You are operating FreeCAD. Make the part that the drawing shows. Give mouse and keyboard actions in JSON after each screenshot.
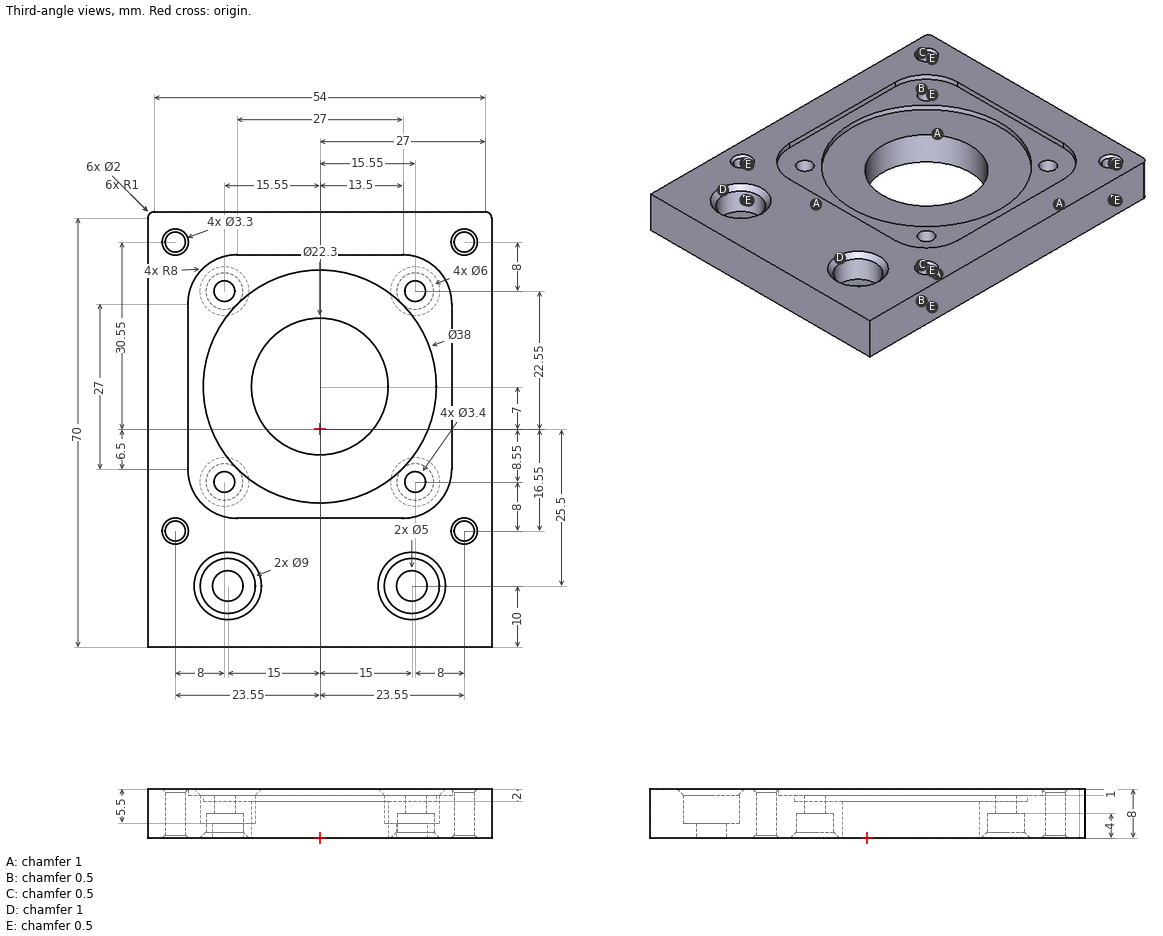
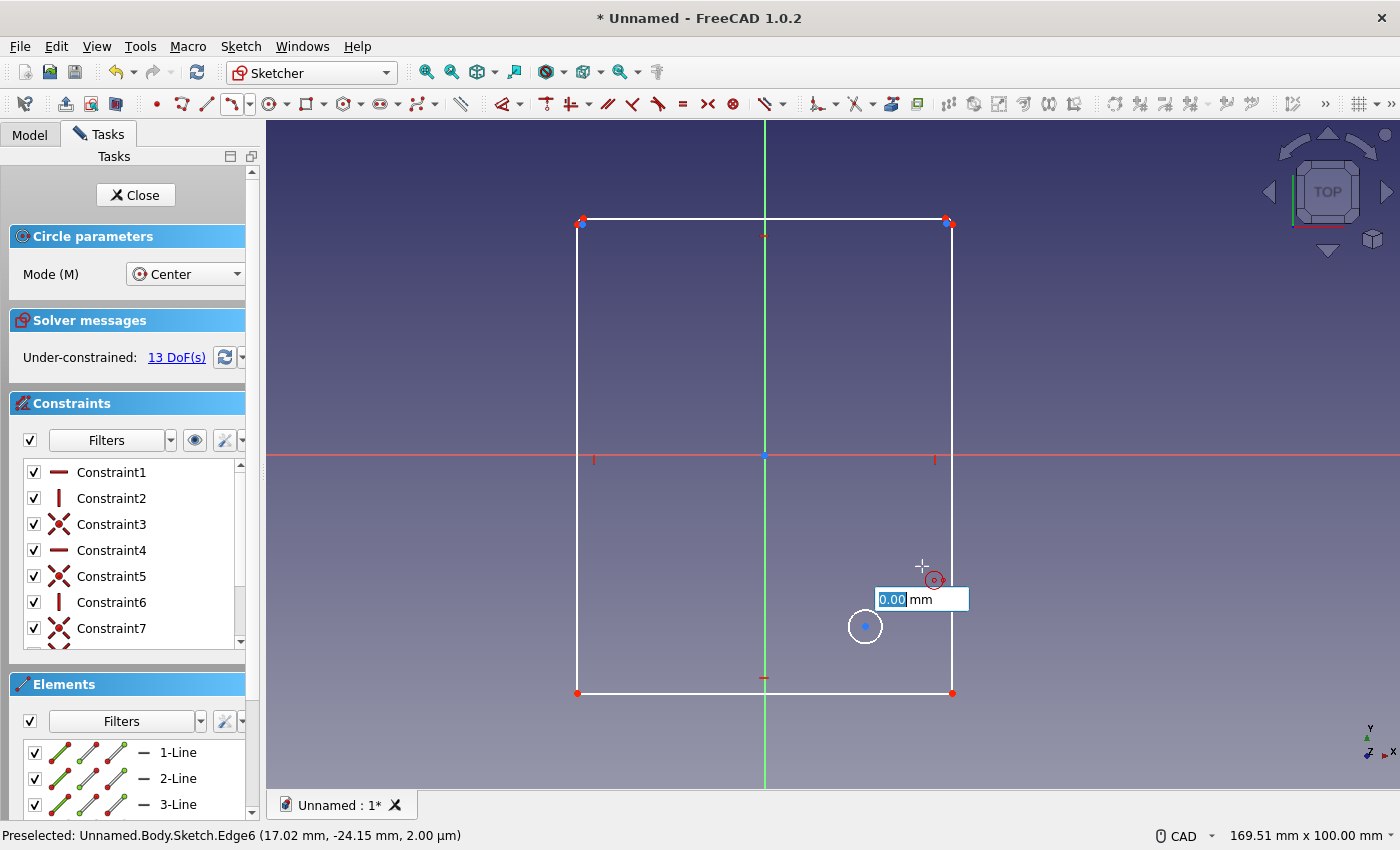
{"action": "scroll", "coordinate": [927, 561], "scroll_direction": "up", "scroll_amount": 5}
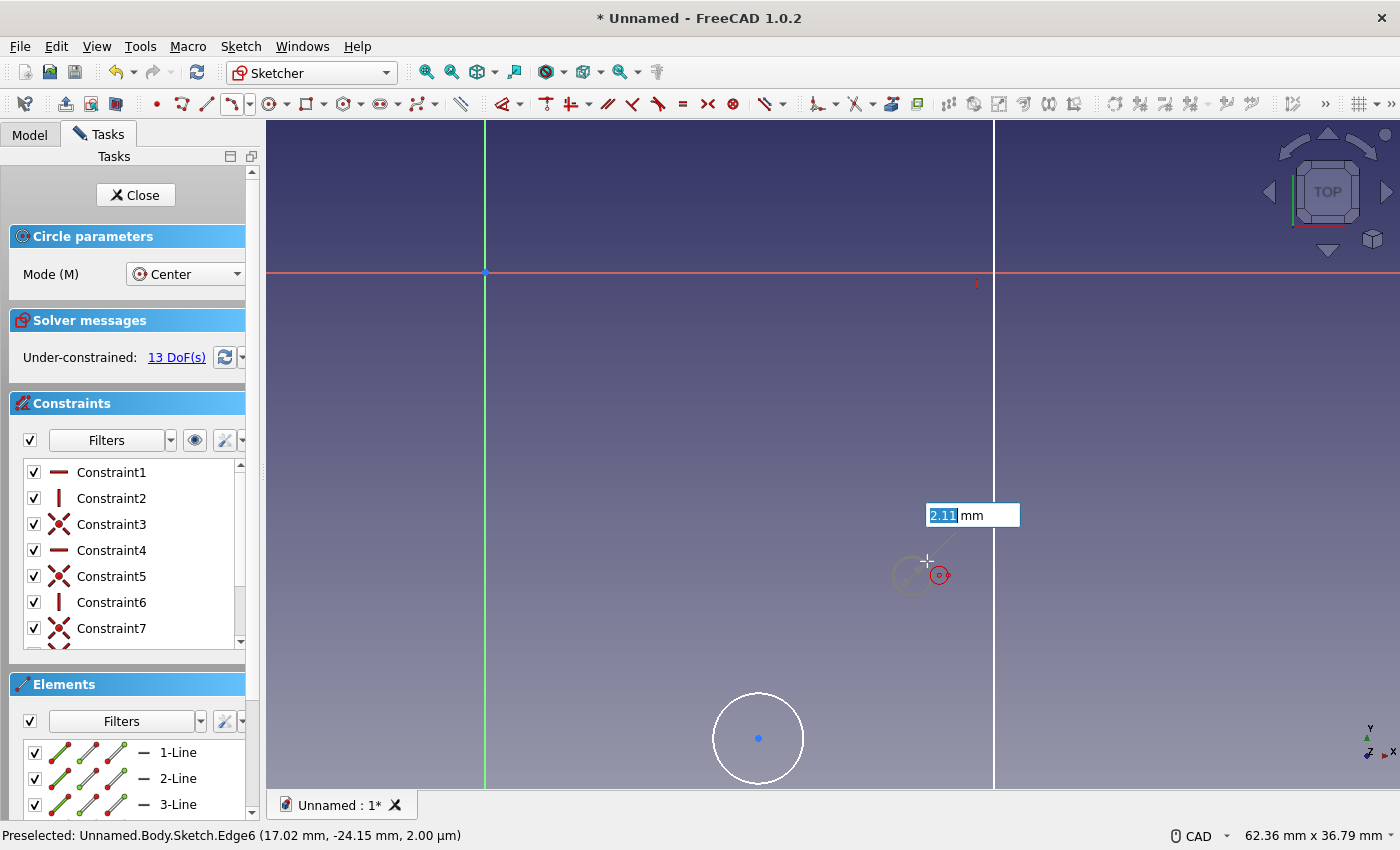
{"action": "left_click", "coordinate": [926, 561]}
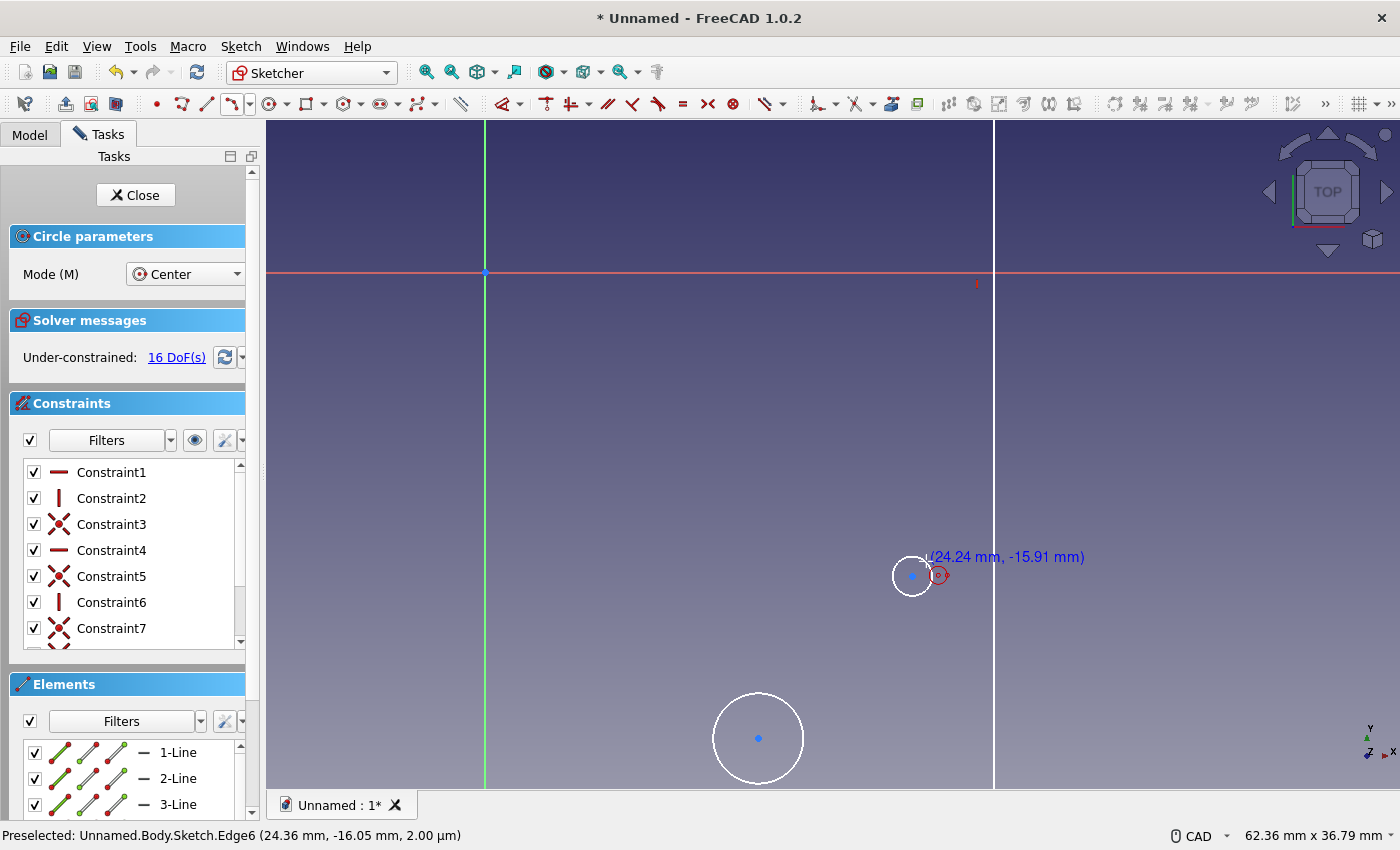
{"action": "left_click", "coordinate": [768, 428]}
{"action": "left_click", "coordinate": [790, 406]}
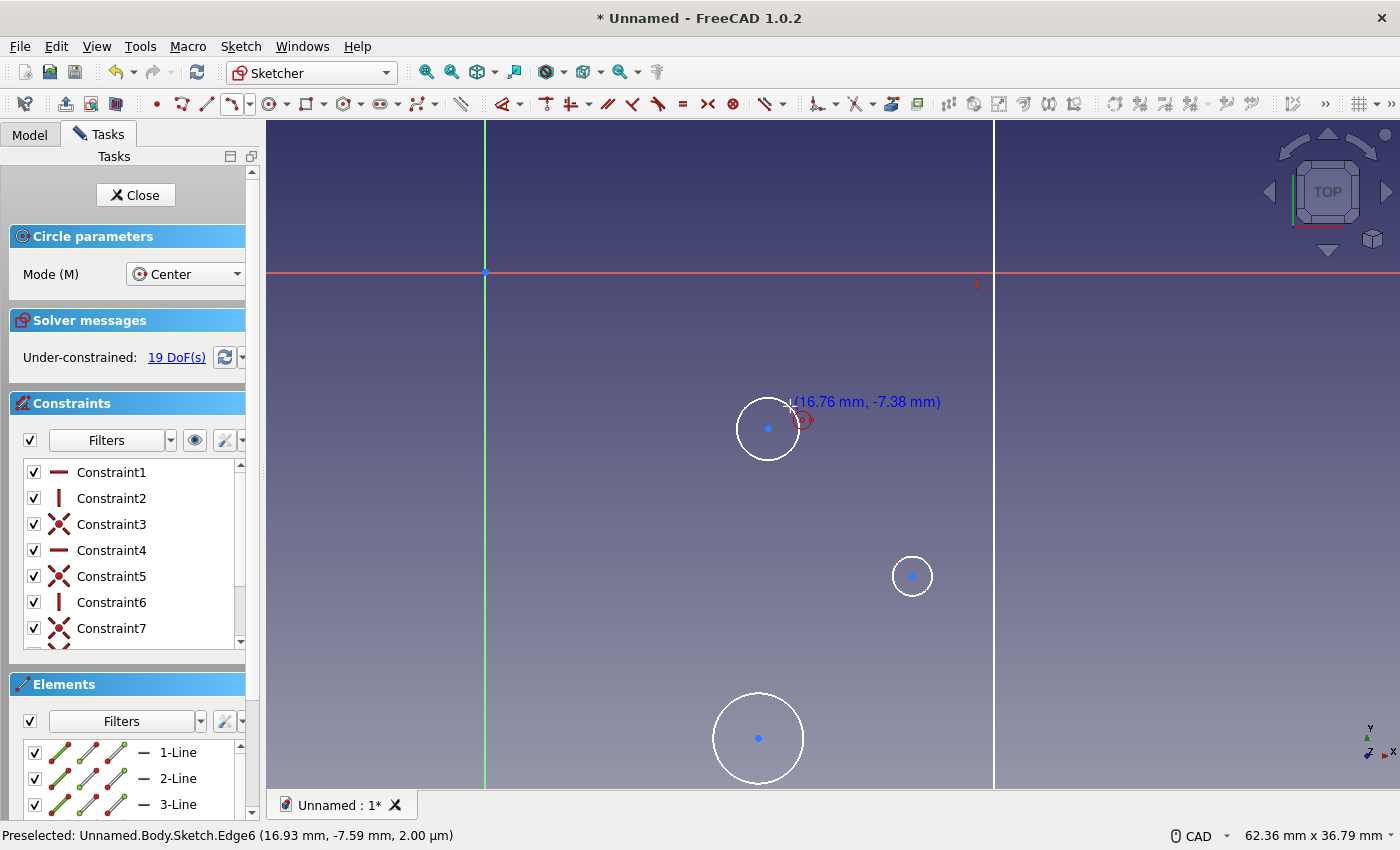
{"action": "scroll", "coordinate": [927, 560], "scroll_direction": "down", "scroll_amount": 5}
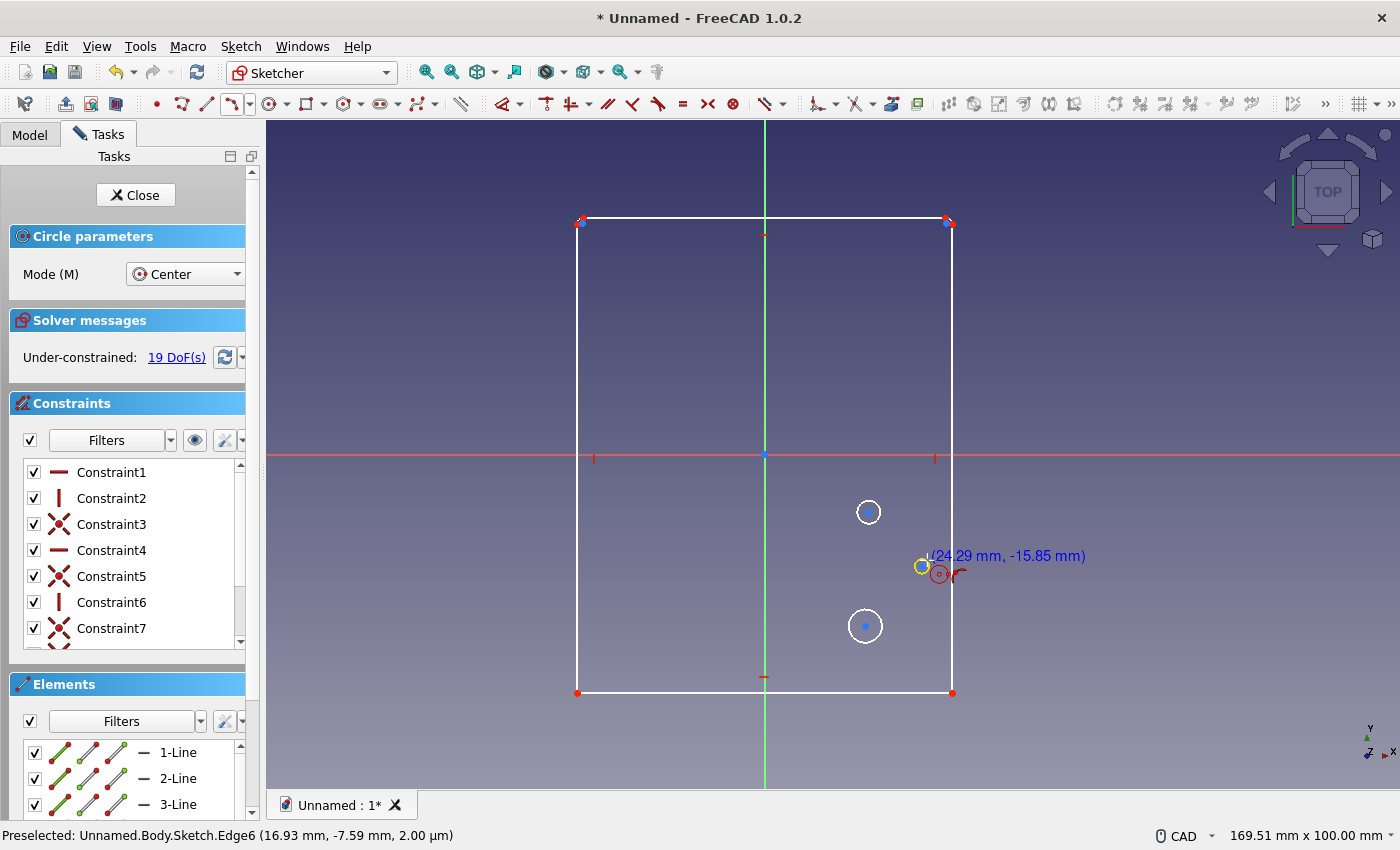
{"action": "scroll", "coordinate": [665, 625], "scroll_direction": "up", "scroll_amount": 2}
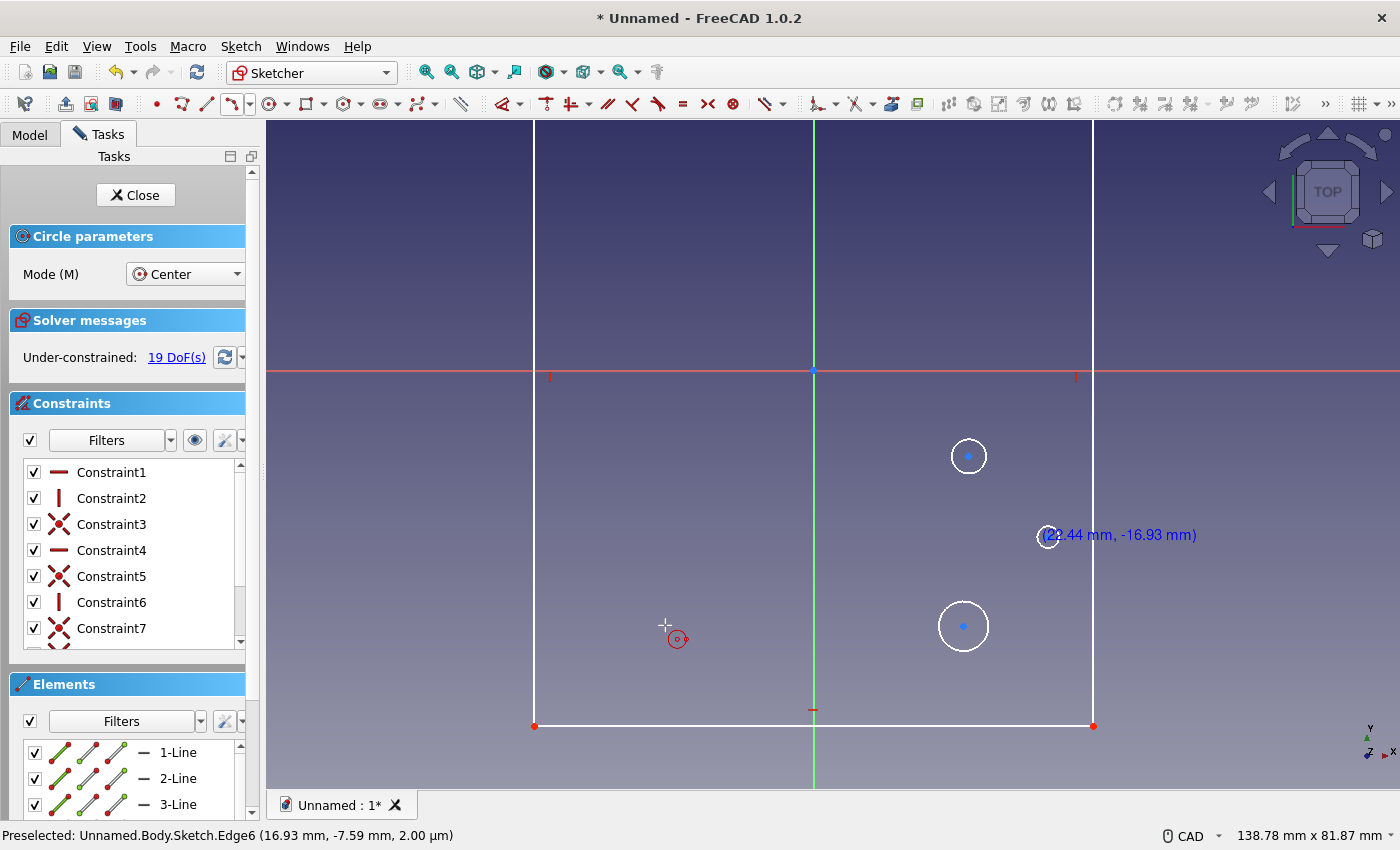
{"action": "left_click", "coordinate": [664, 625]}
{"action": "left_click", "coordinate": [682, 607]}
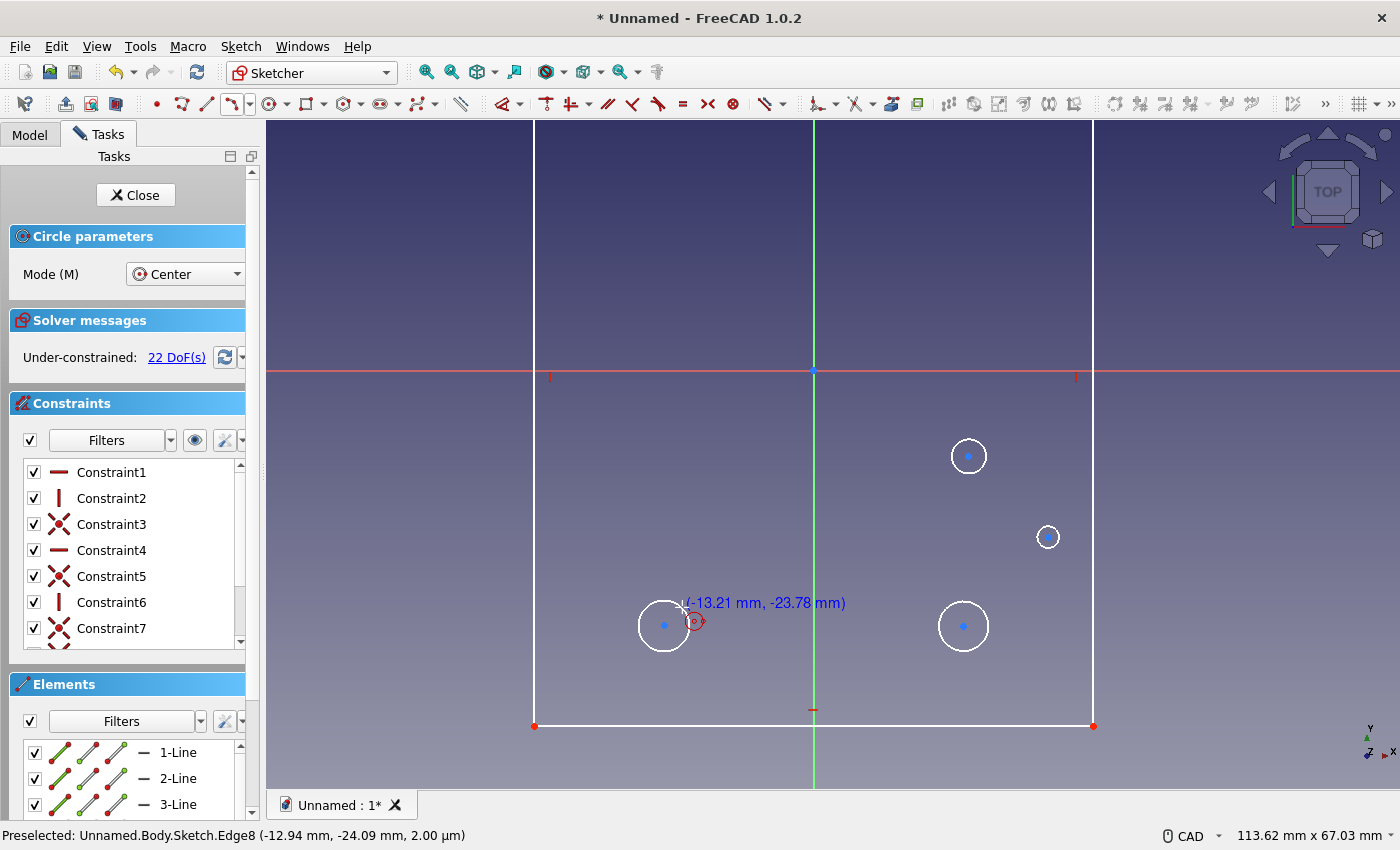
{"action": "scroll", "coordinate": [579, 536], "scroll_direction": "up", "scroll_amount": 5}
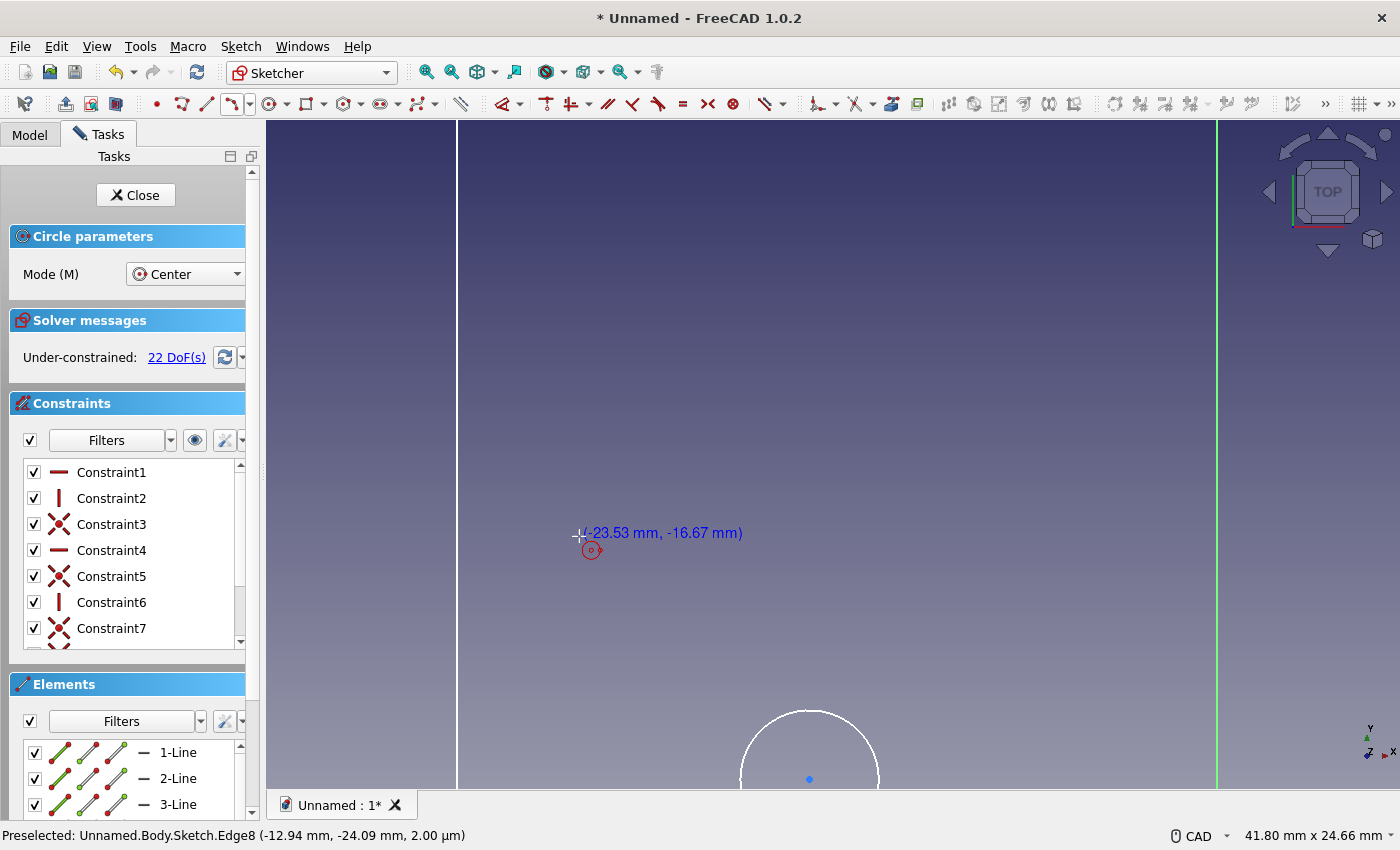
{"action": "scroll", "coordinate": [616, 575], "scroll_direction": "down", "scroll_amount": 7}